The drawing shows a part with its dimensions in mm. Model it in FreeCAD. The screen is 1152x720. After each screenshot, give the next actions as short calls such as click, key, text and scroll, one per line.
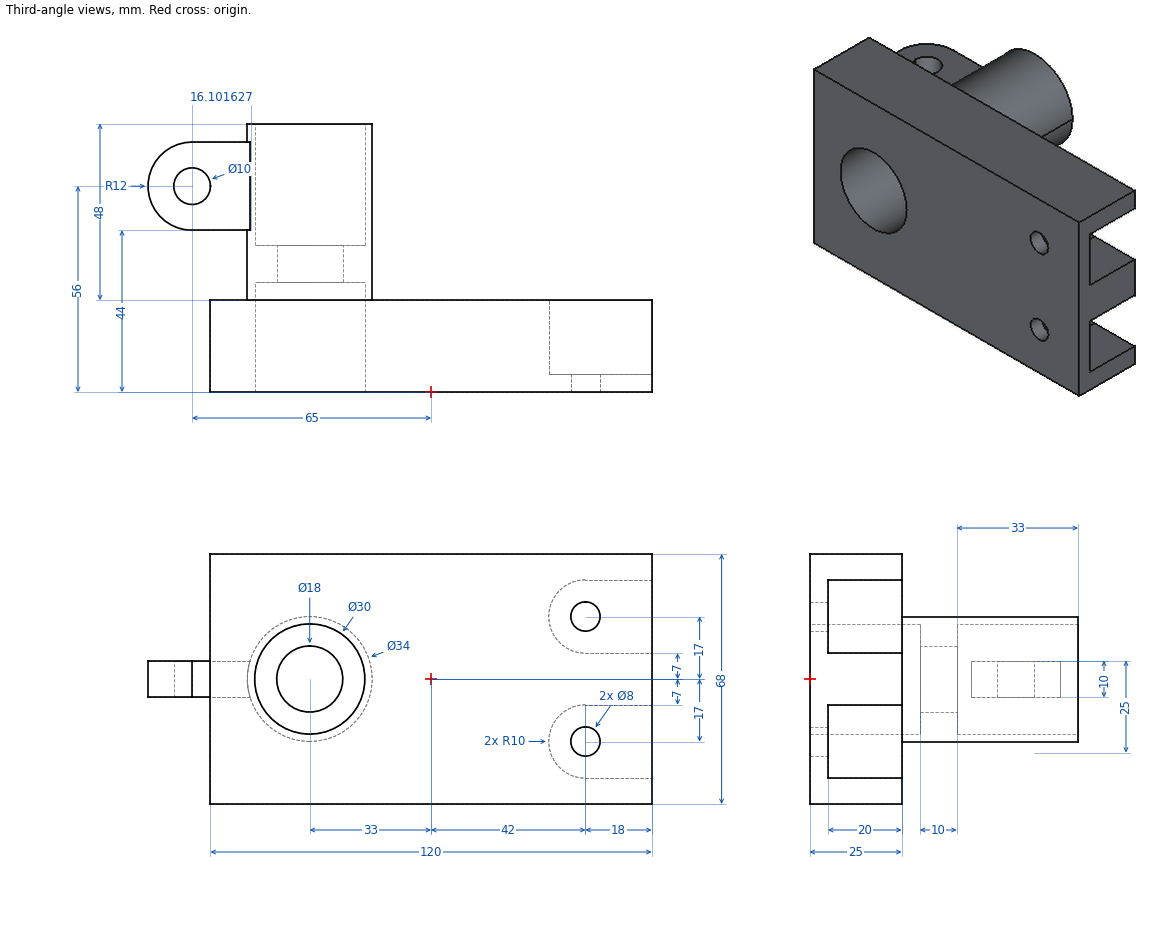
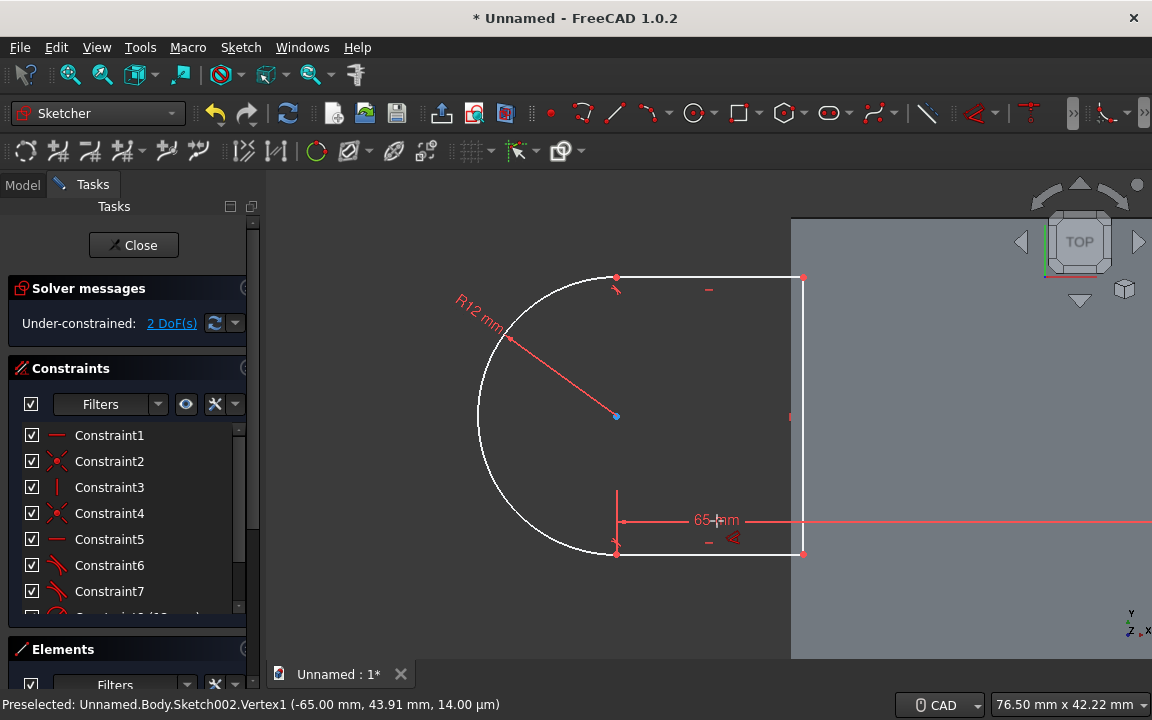
click(617, 555)
click(583, 593)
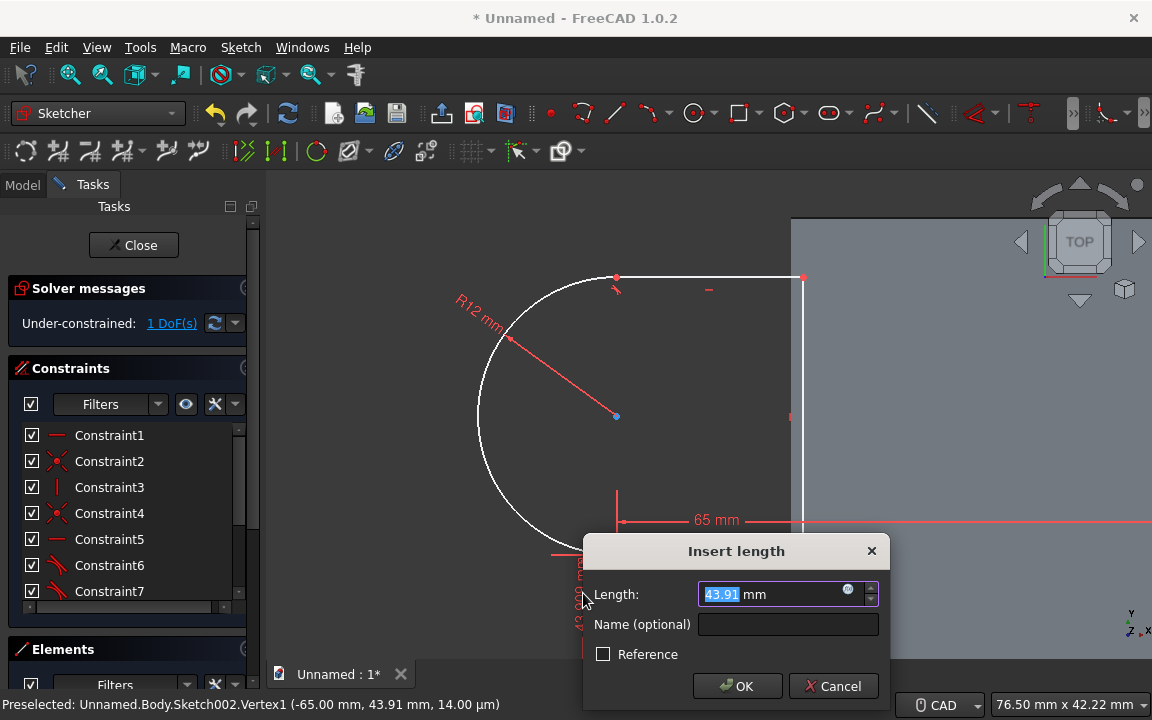
text(44)
key(Return)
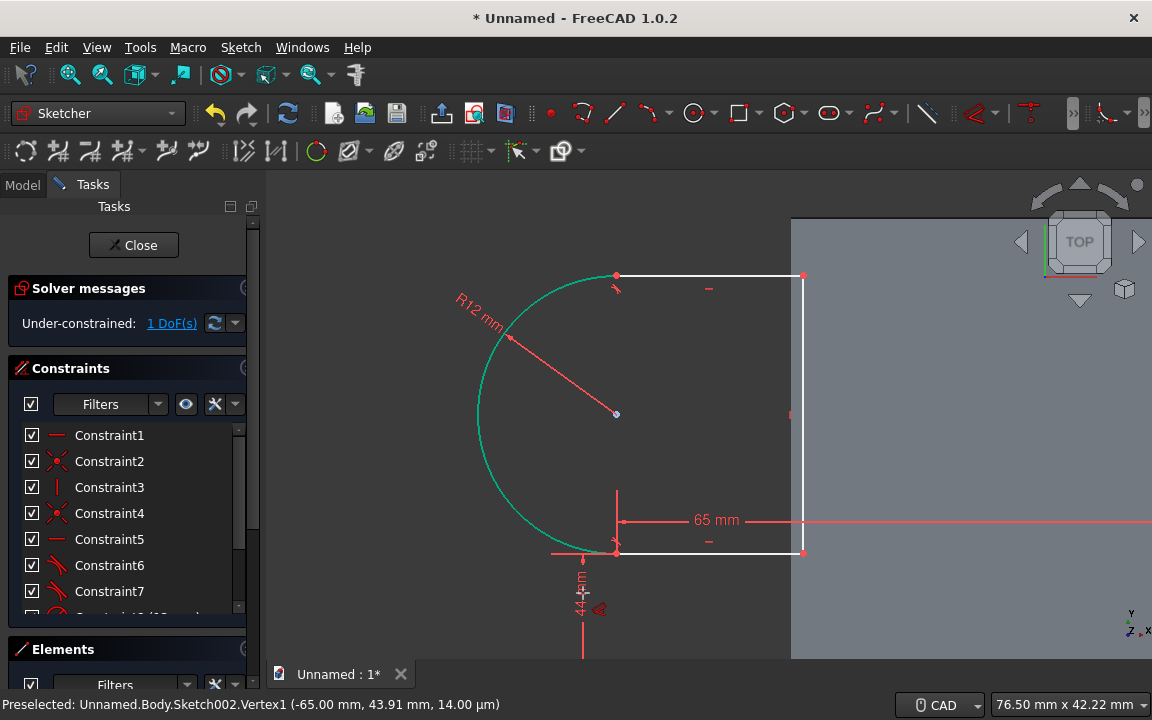
click(673, 554)
click(710, 588)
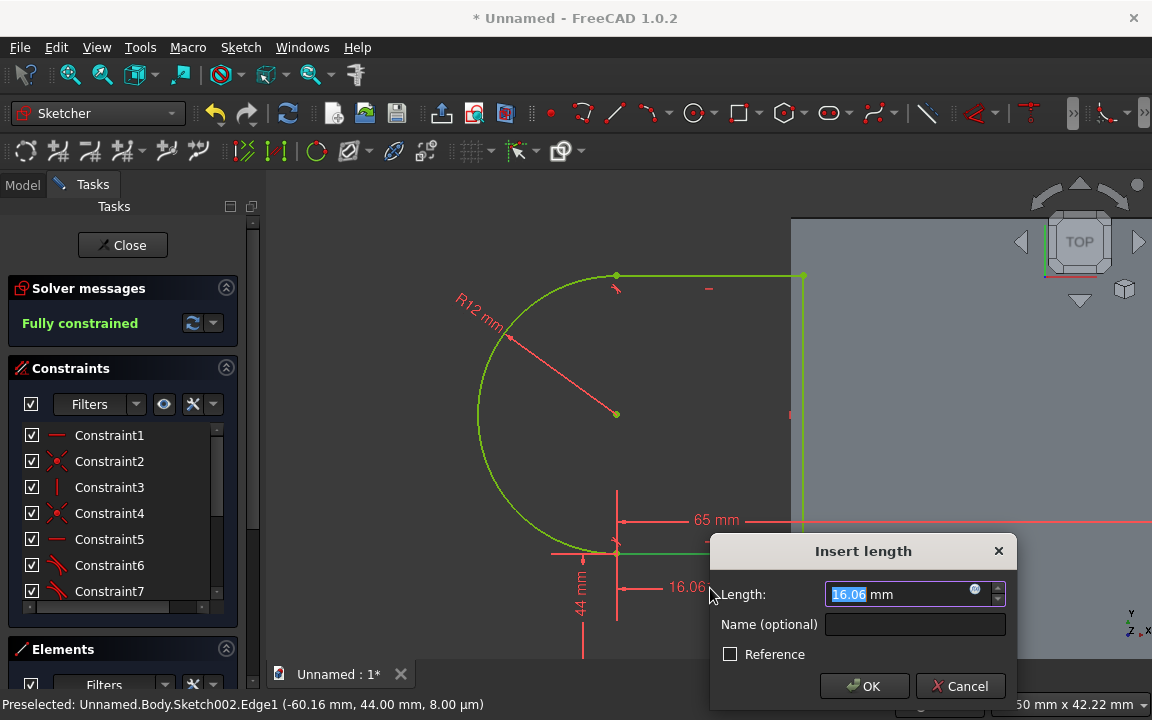
text(16.101627)
key(Return)
key(Escape)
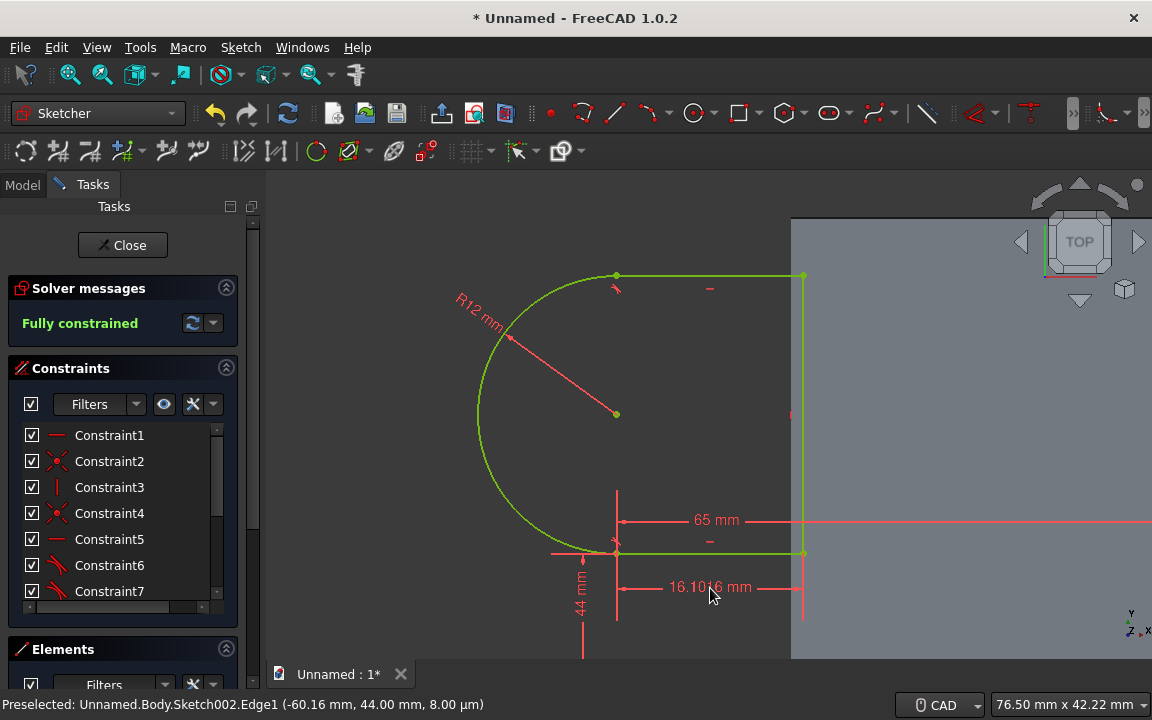
click(123, 245)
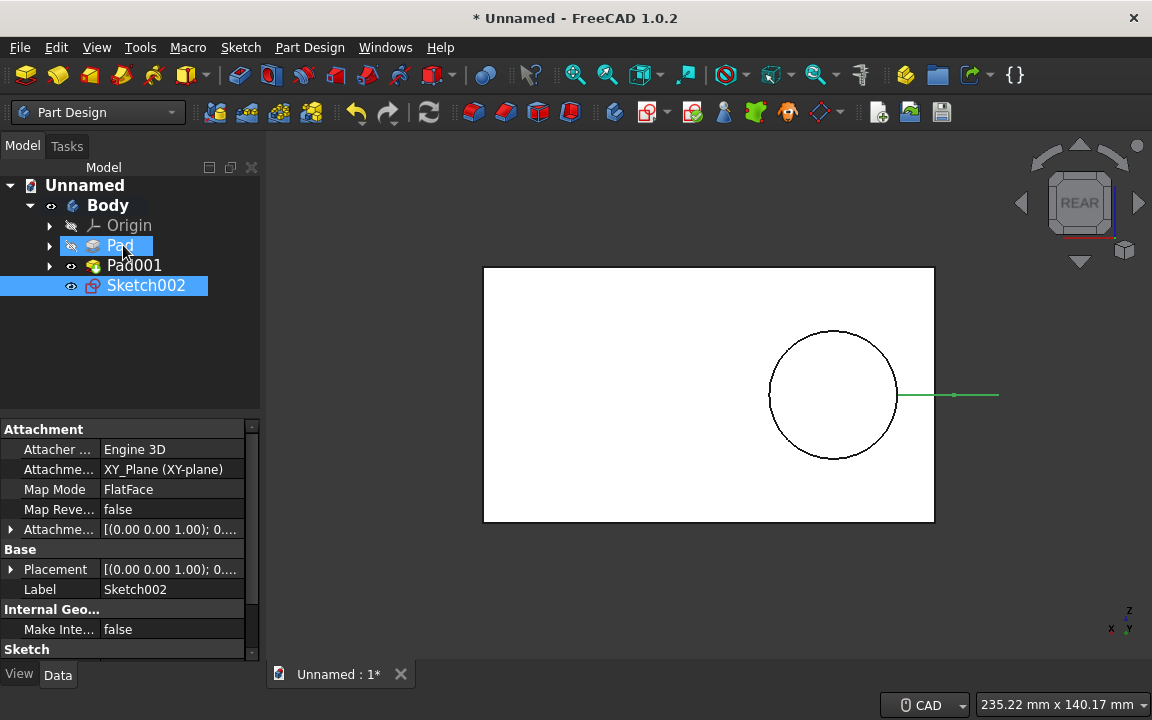
click(26, 76)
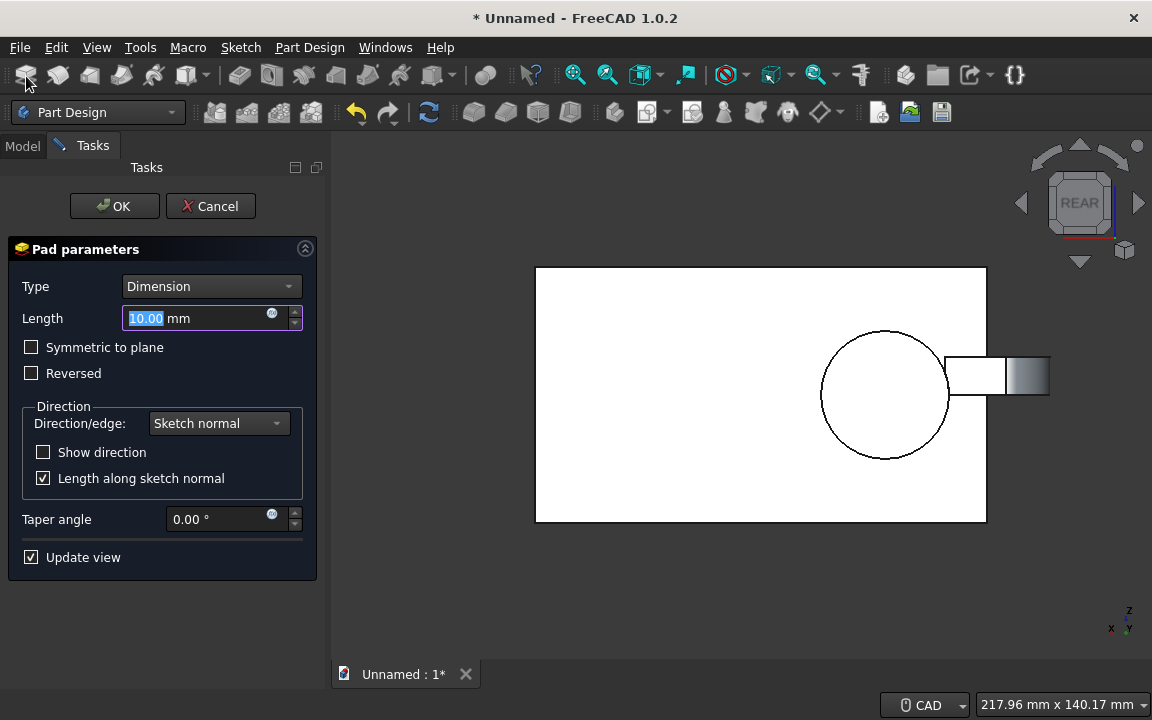
text(10)
key(Tab)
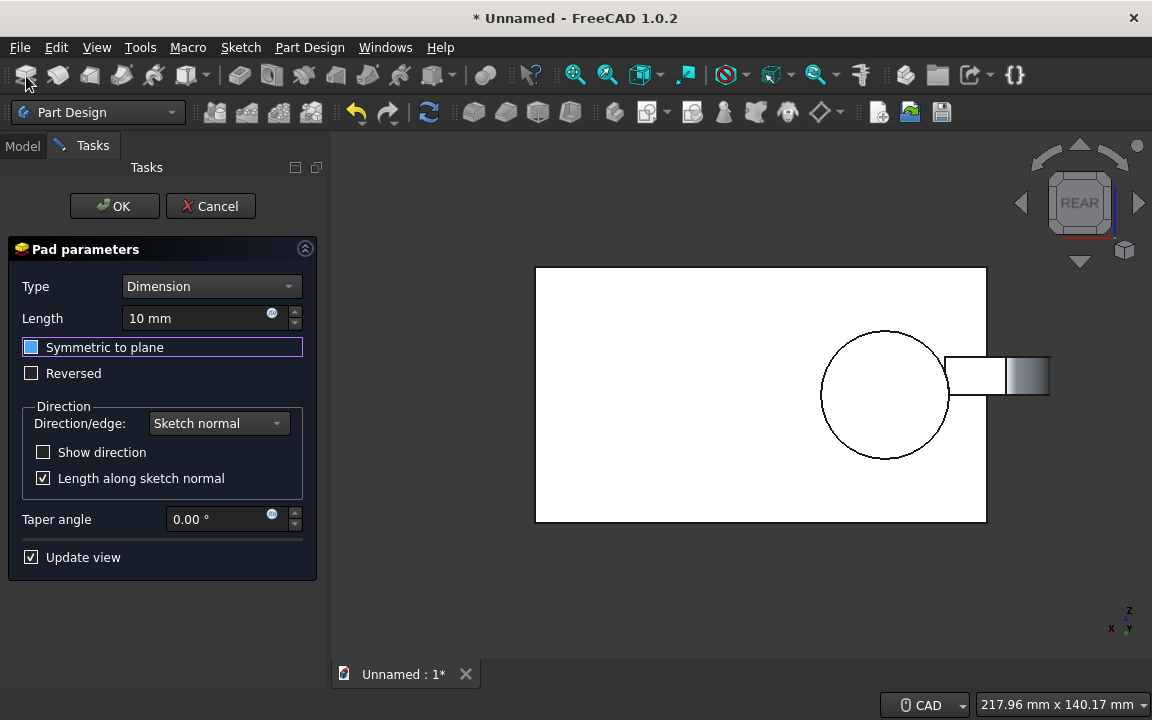
click(30, 347)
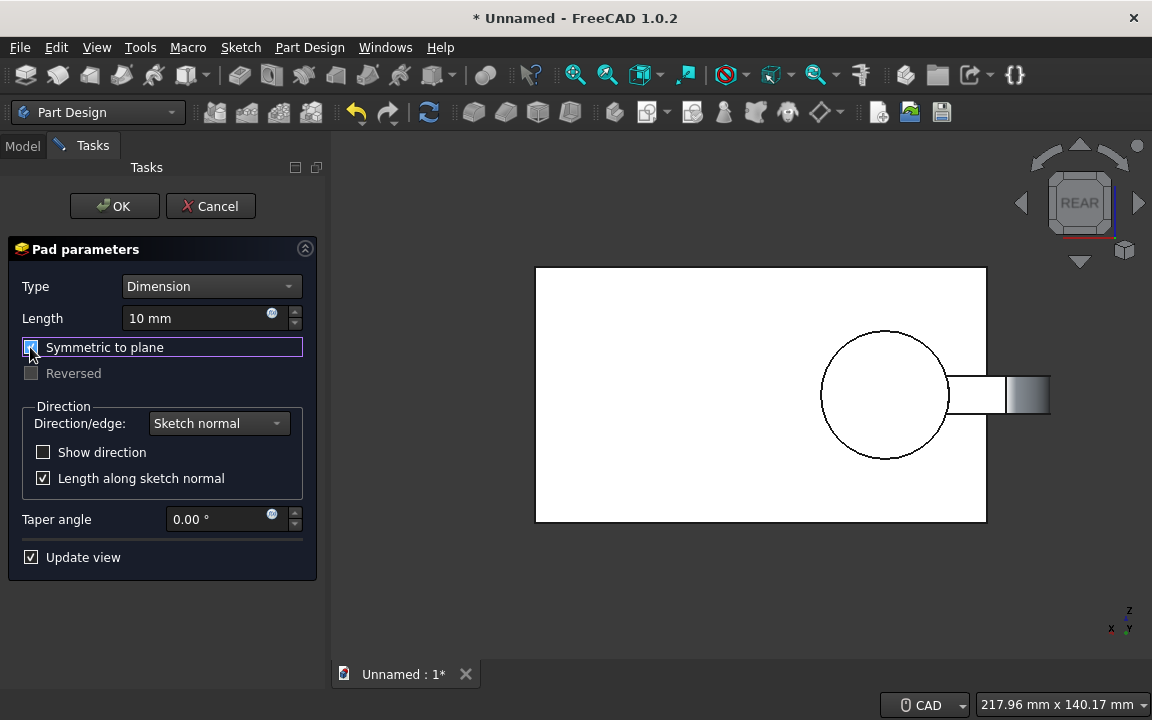
click(115, 206)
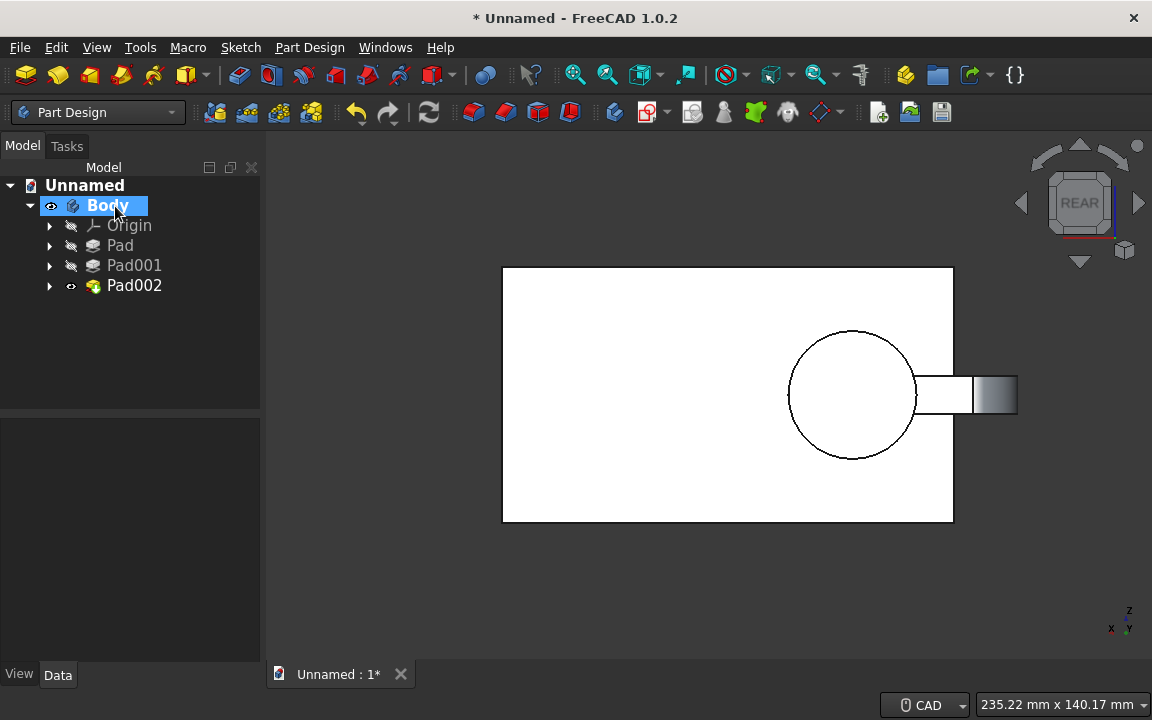
click(853, 394)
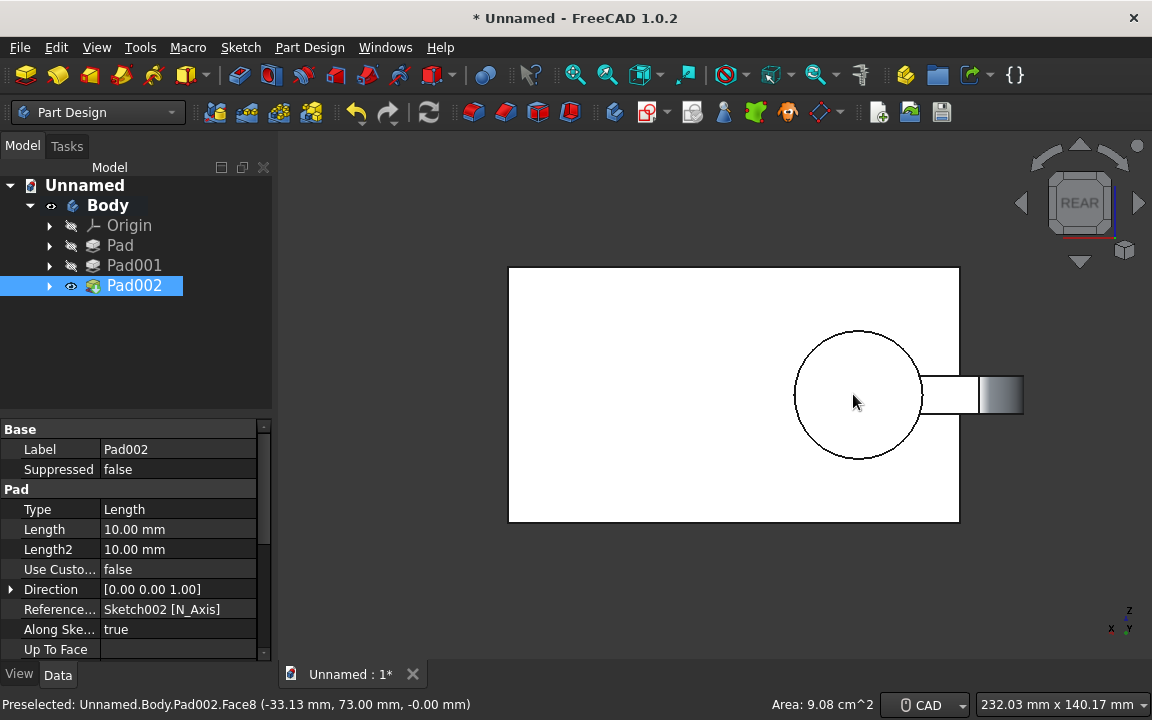
click(648, 112)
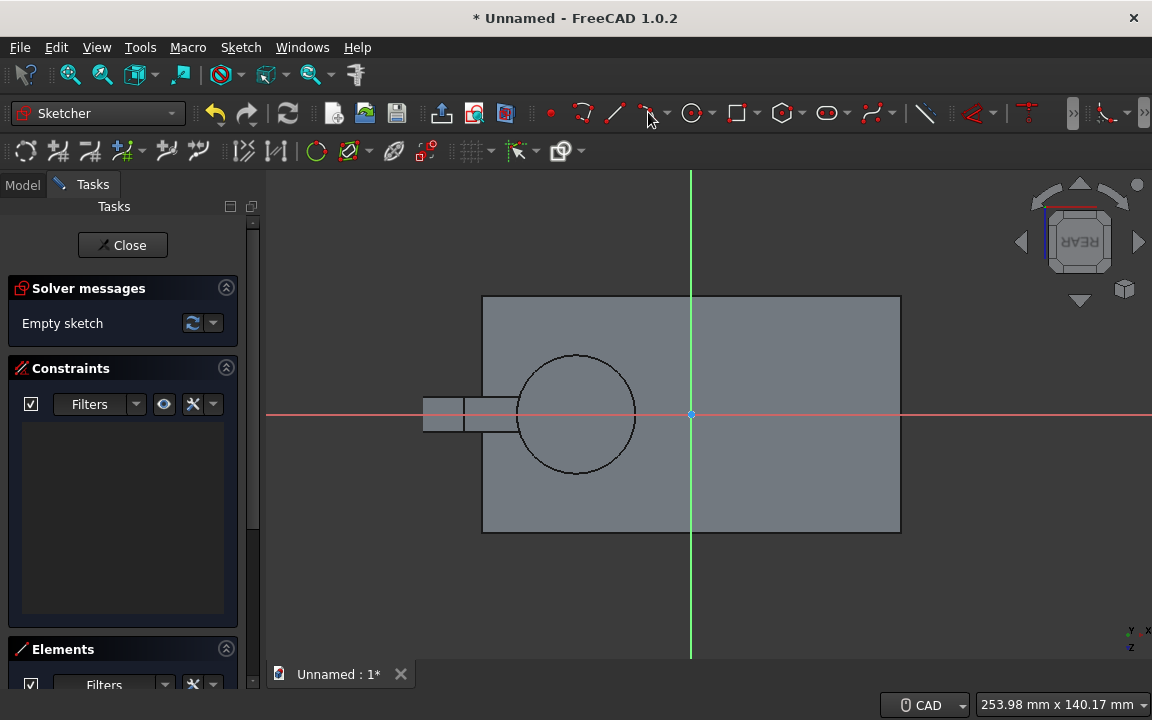
scroll(588, 414, up, 5)